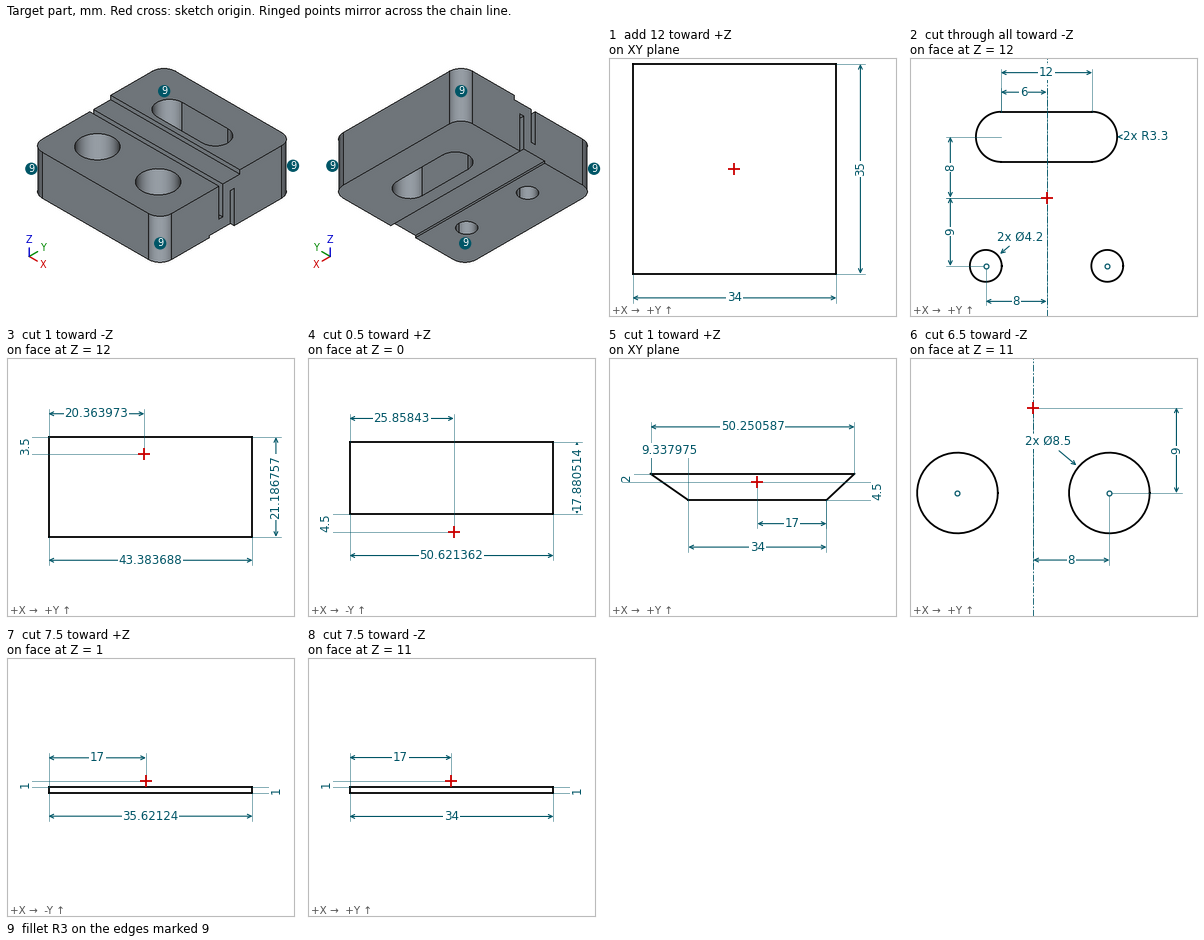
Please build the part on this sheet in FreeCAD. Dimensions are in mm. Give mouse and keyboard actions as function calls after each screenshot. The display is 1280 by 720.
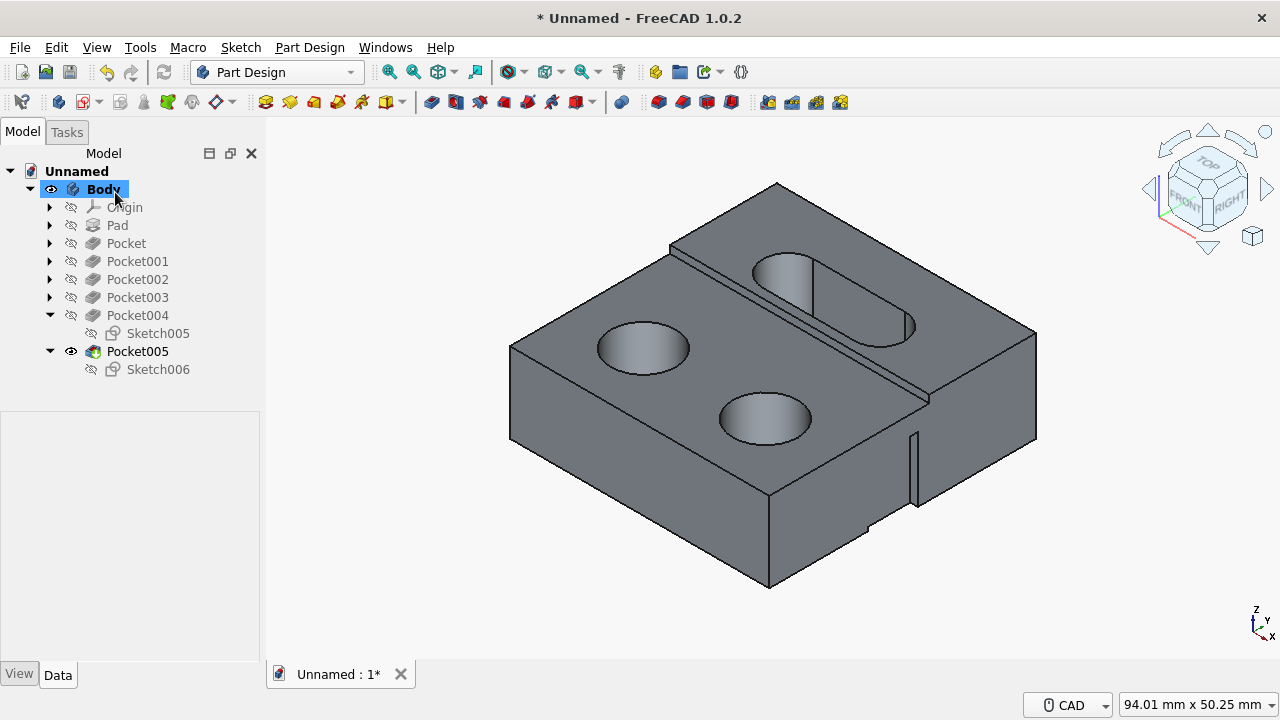
click(742, 361)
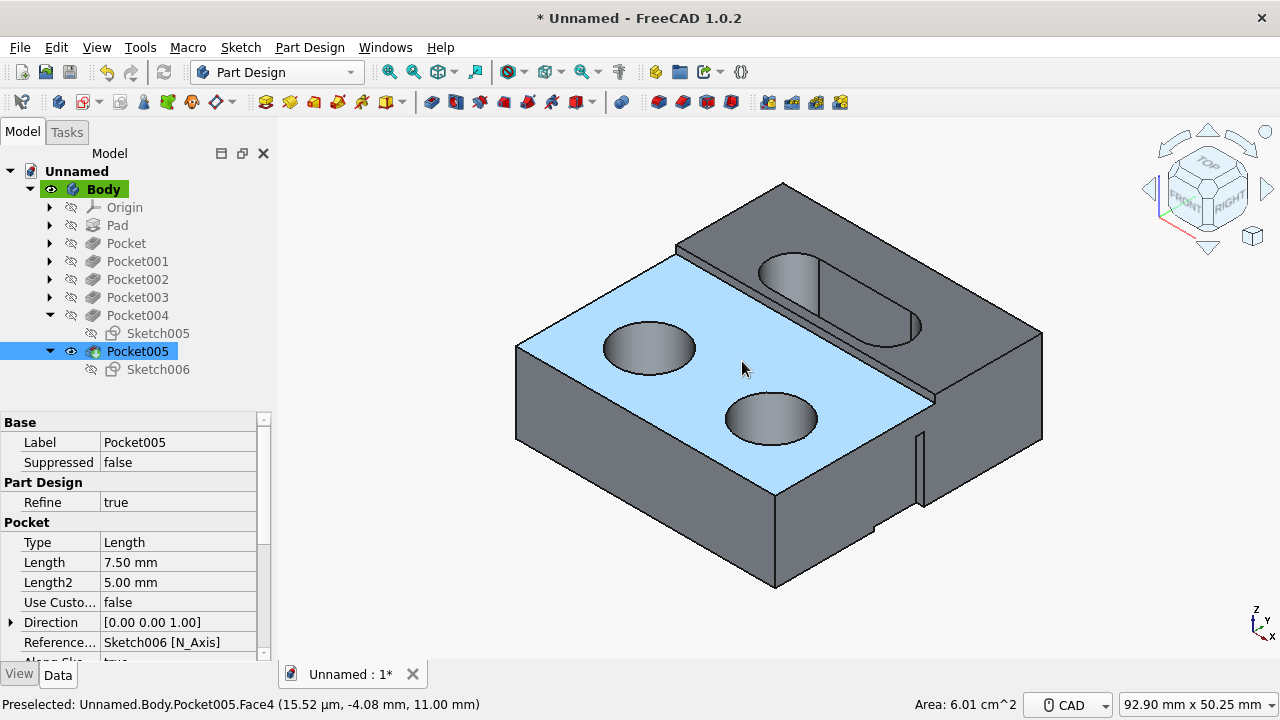
click(84, 102)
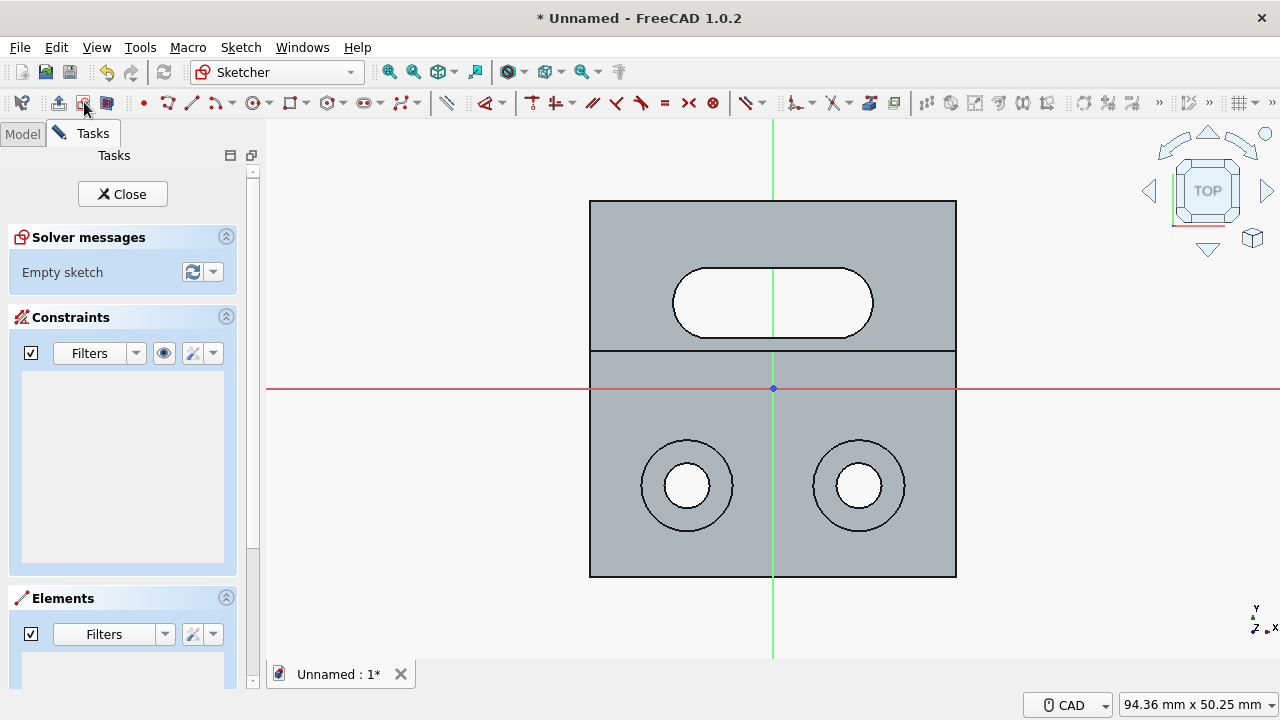
scroll(912, 422, up, 2)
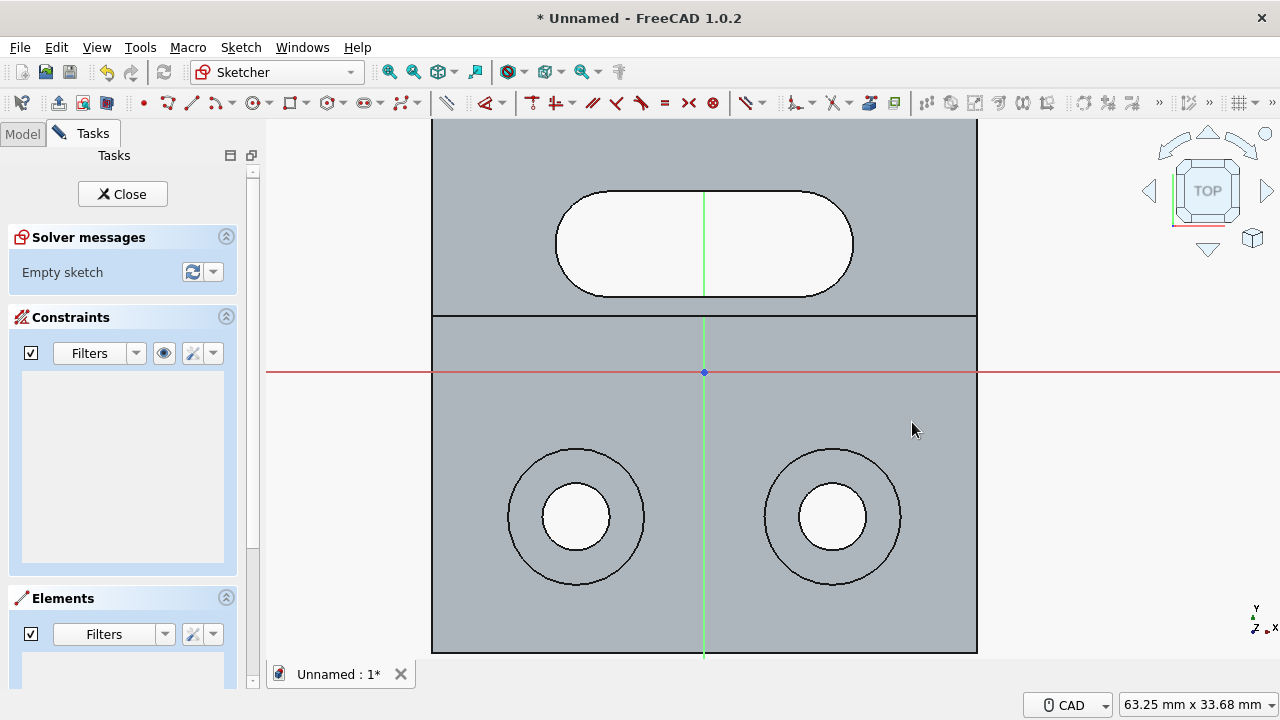
key(g)
key(r)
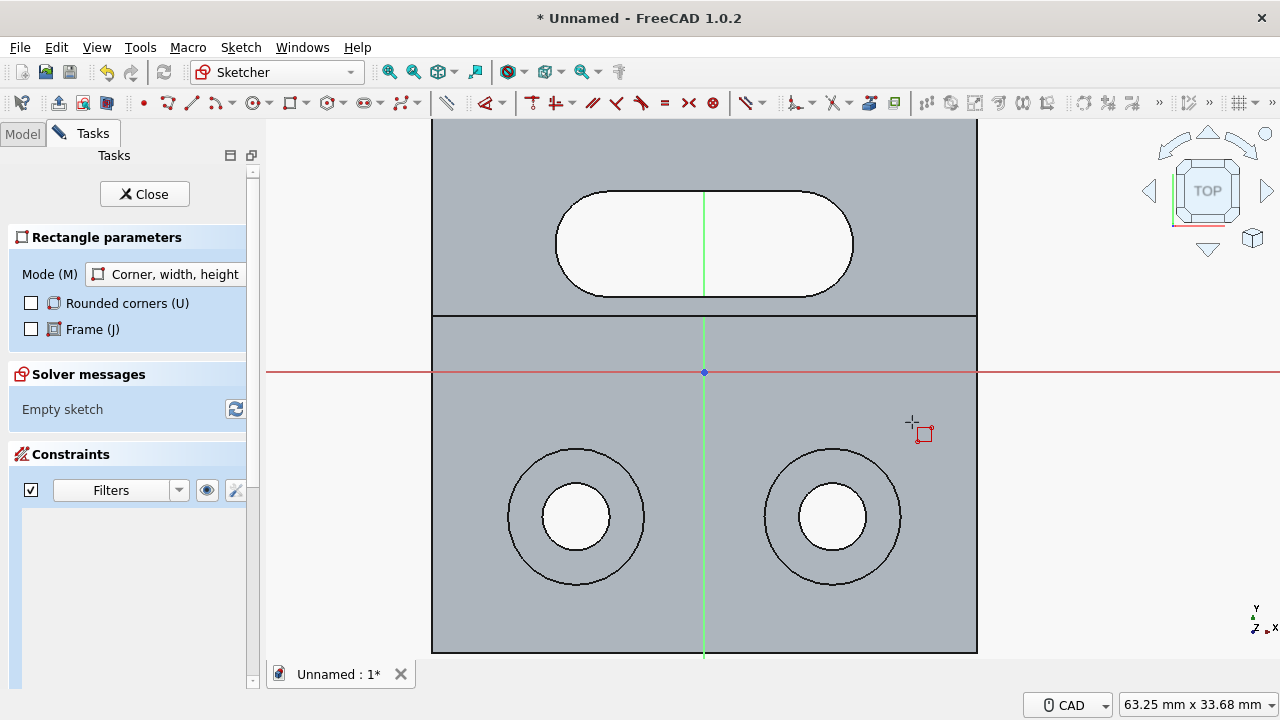
click(432, 389)
move(977, 405)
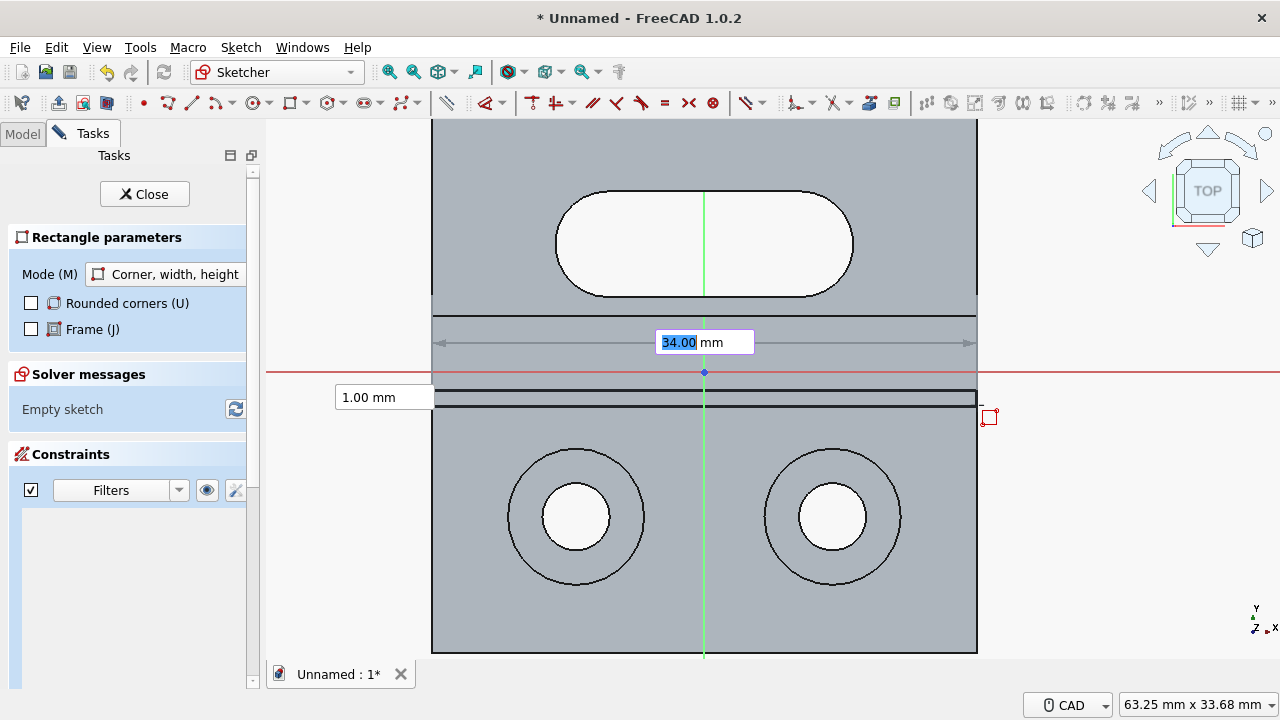
text(34)
key(Tab)
text(1)
key(Return)
key(Escape)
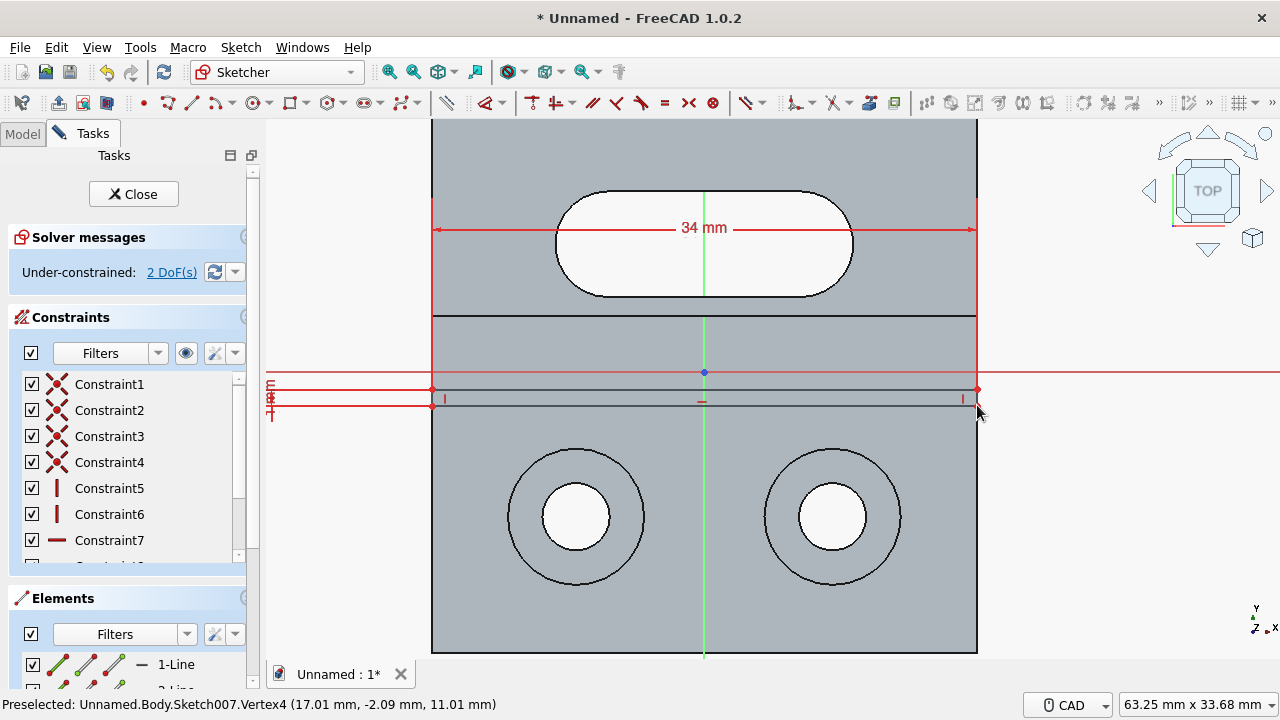
click(486, 104)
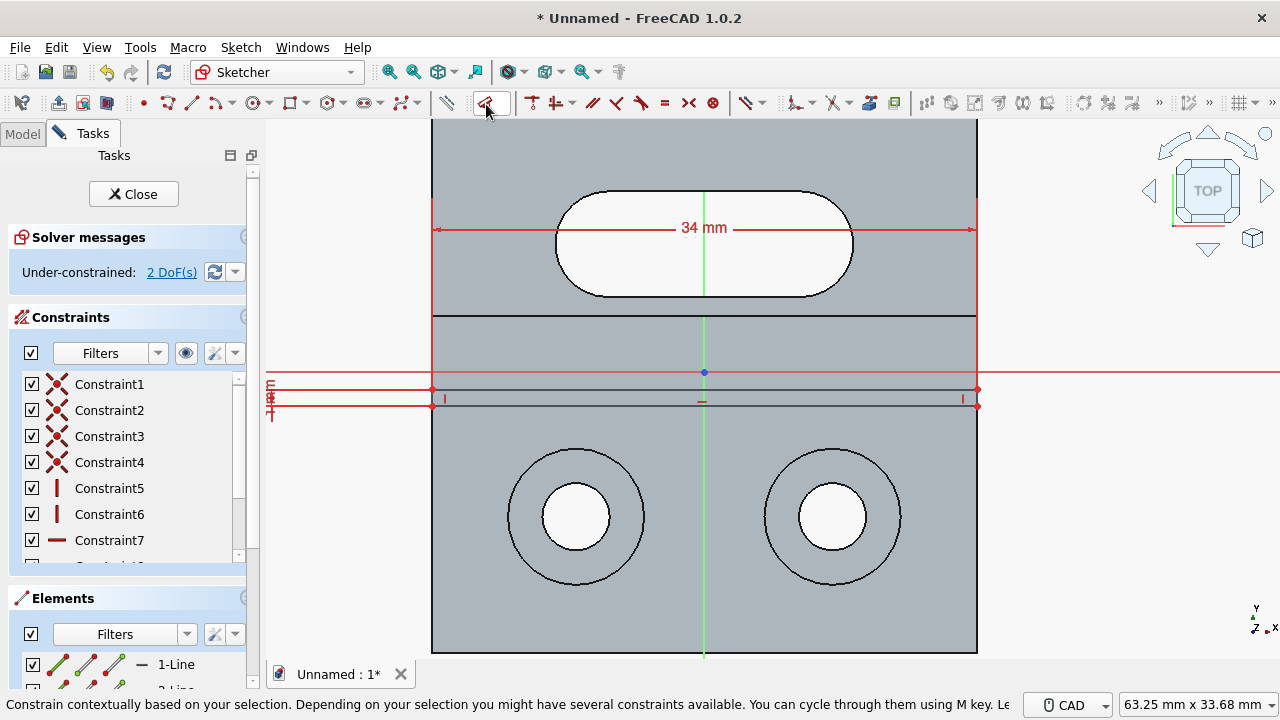
scroll(432, 390, up, 5)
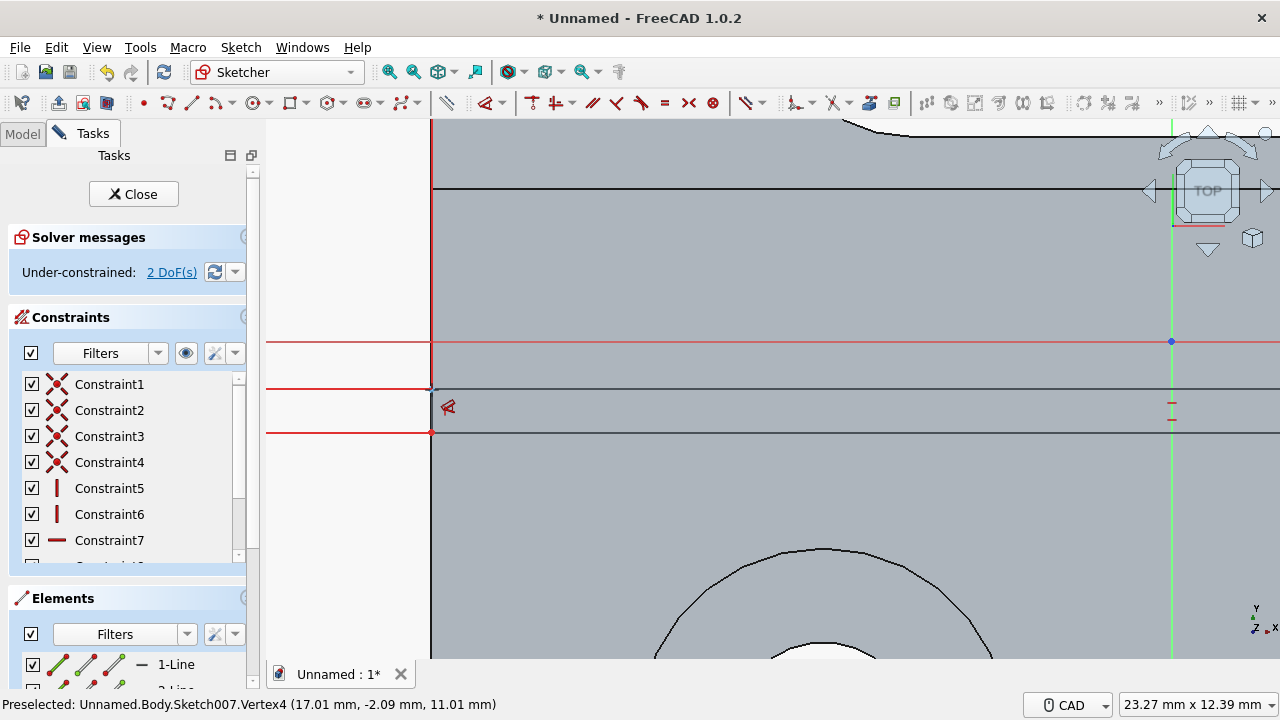
click(432, 389)
click(398, 365)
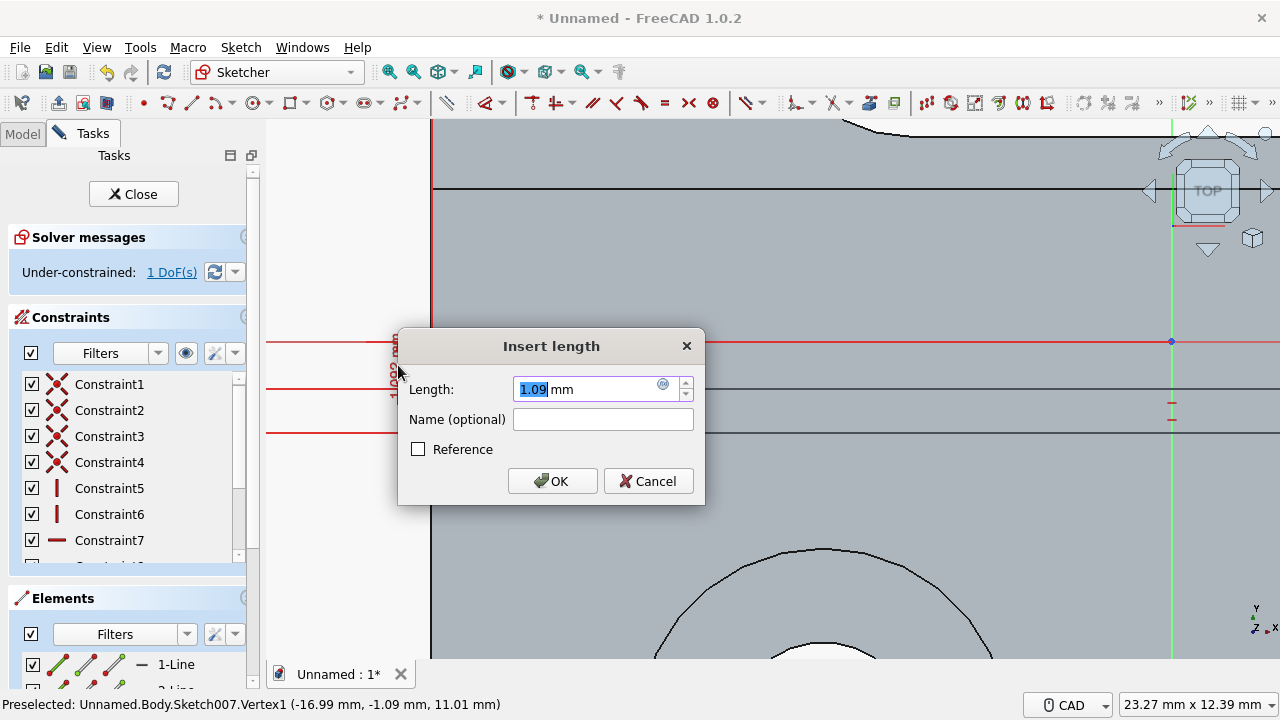
text(1)
key(Return)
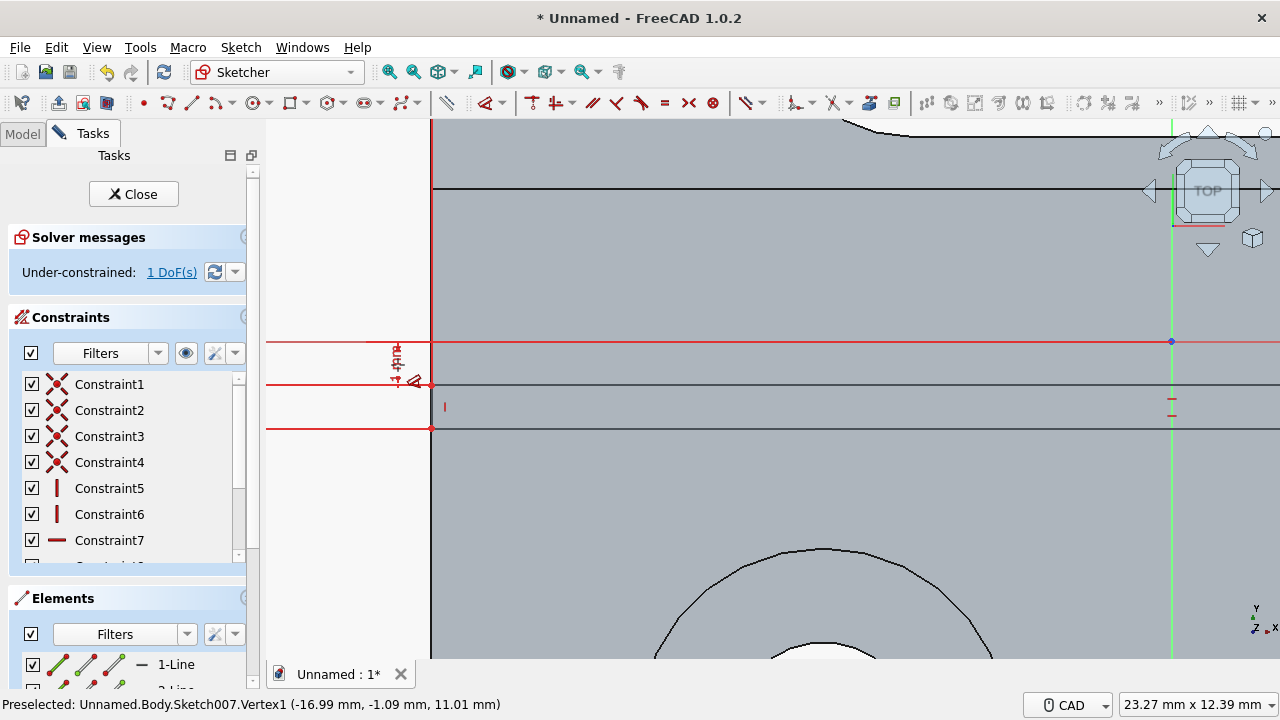
click(432, 385)
click(773, 308)